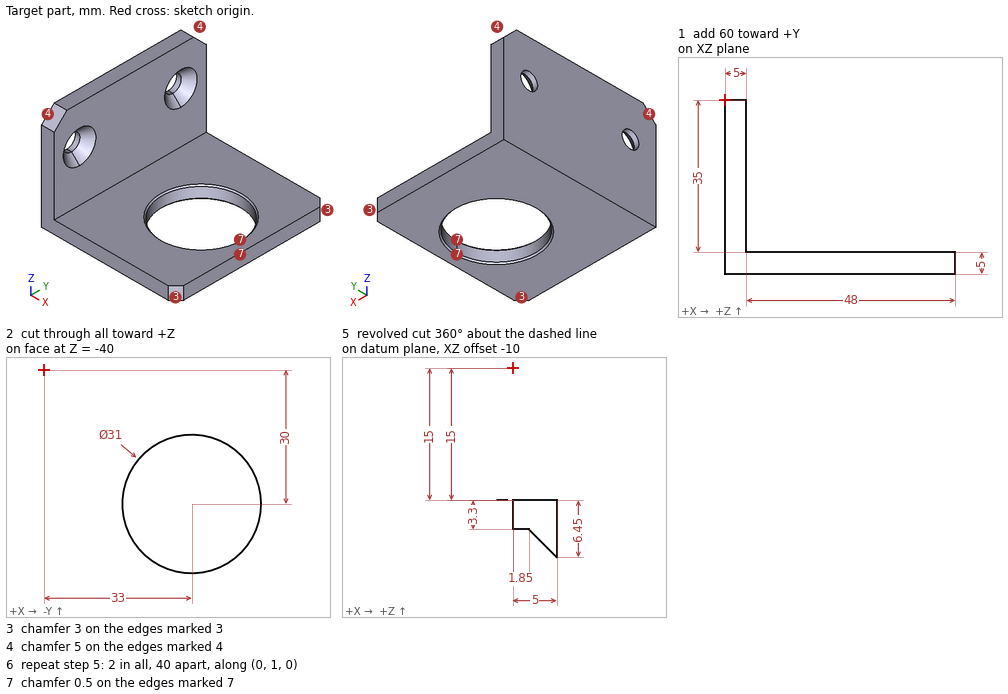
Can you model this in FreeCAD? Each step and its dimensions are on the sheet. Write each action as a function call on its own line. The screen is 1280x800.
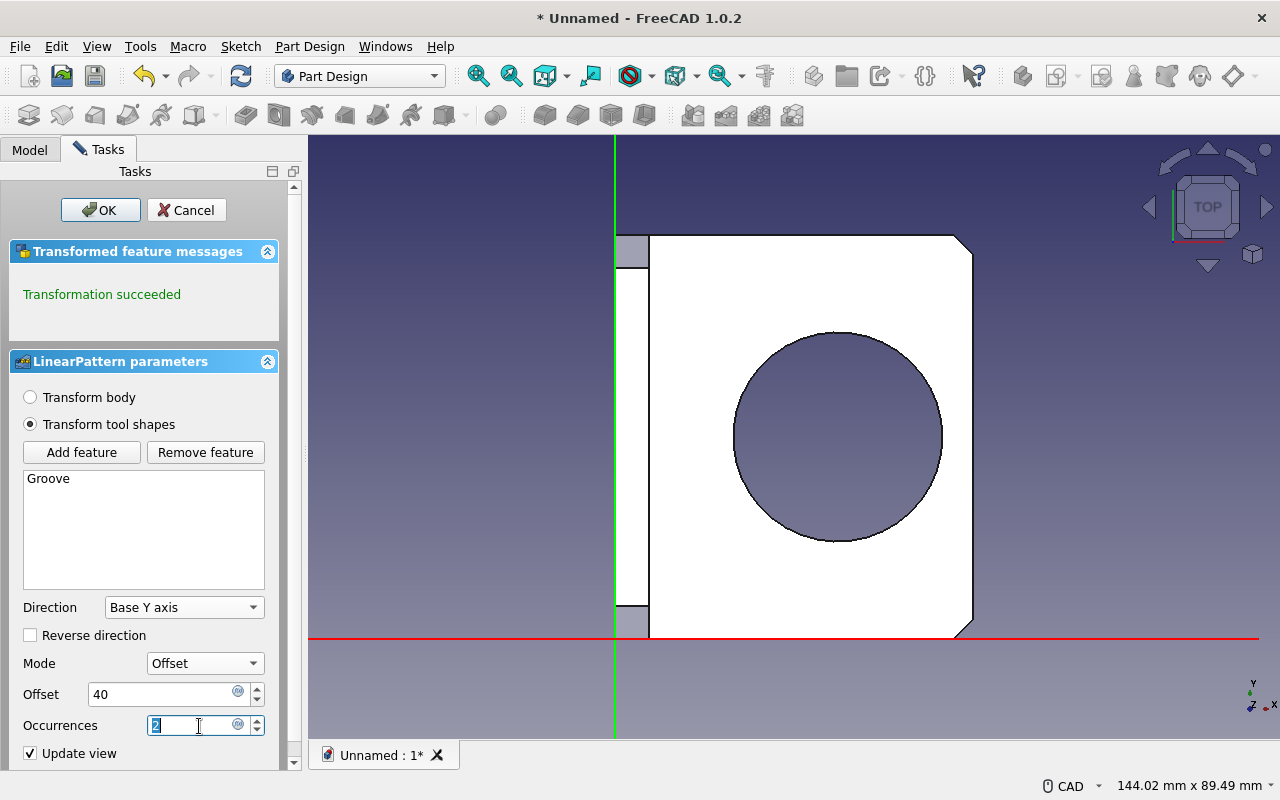
text(2)
key(Tab)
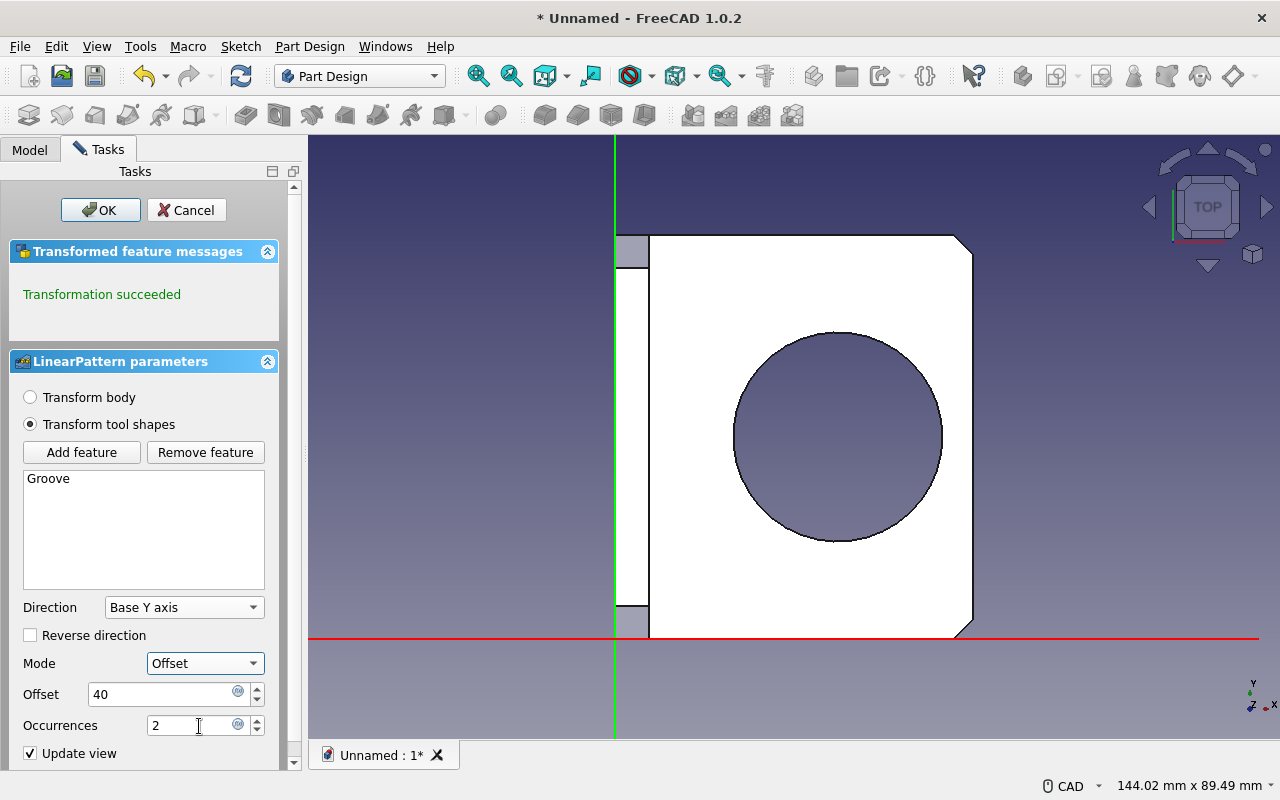
click(101, 210)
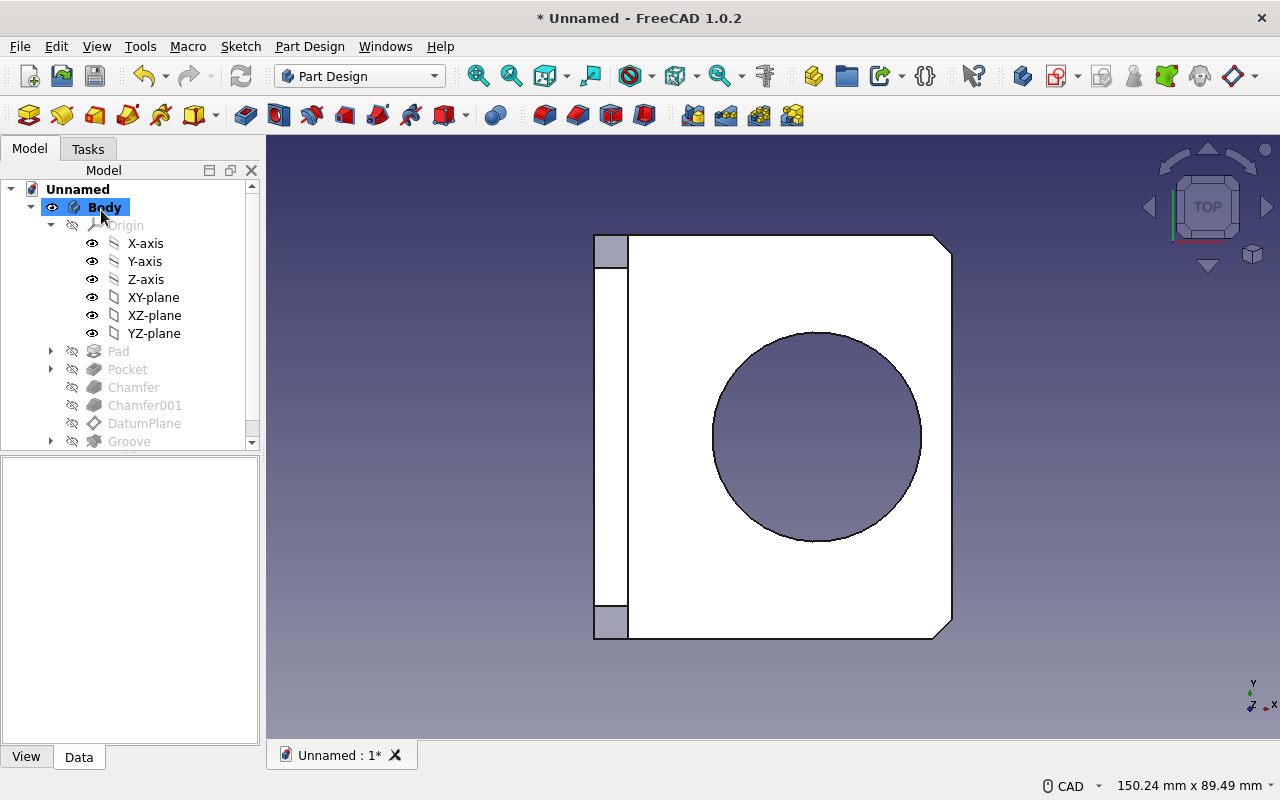
click(712, 436)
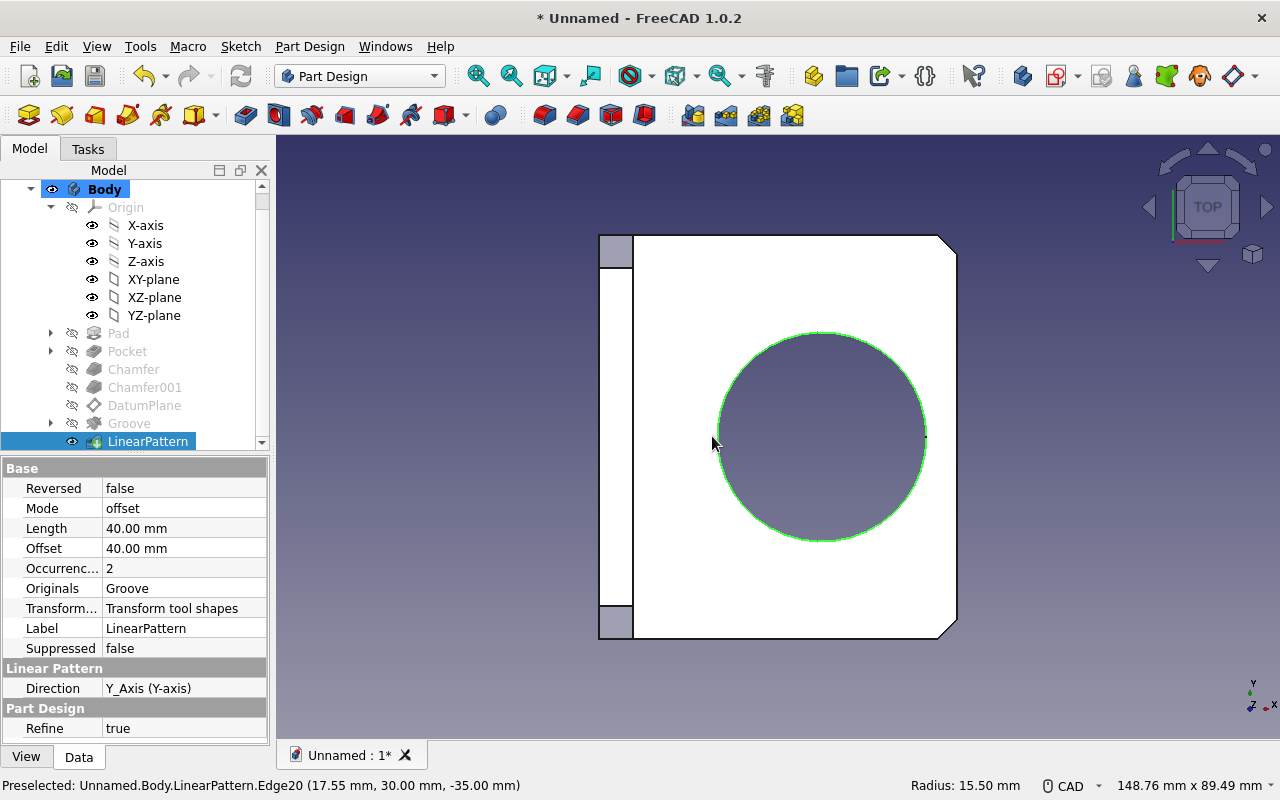
key(0)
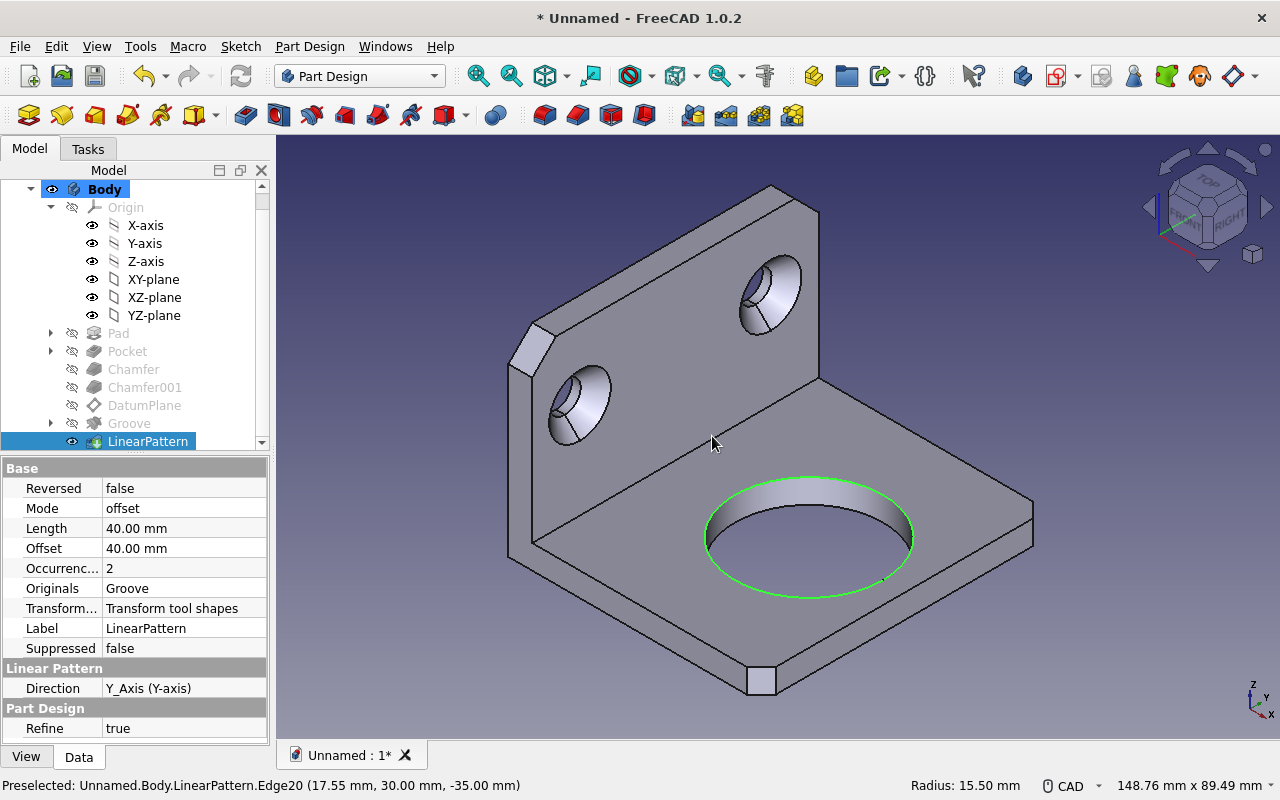
key(2)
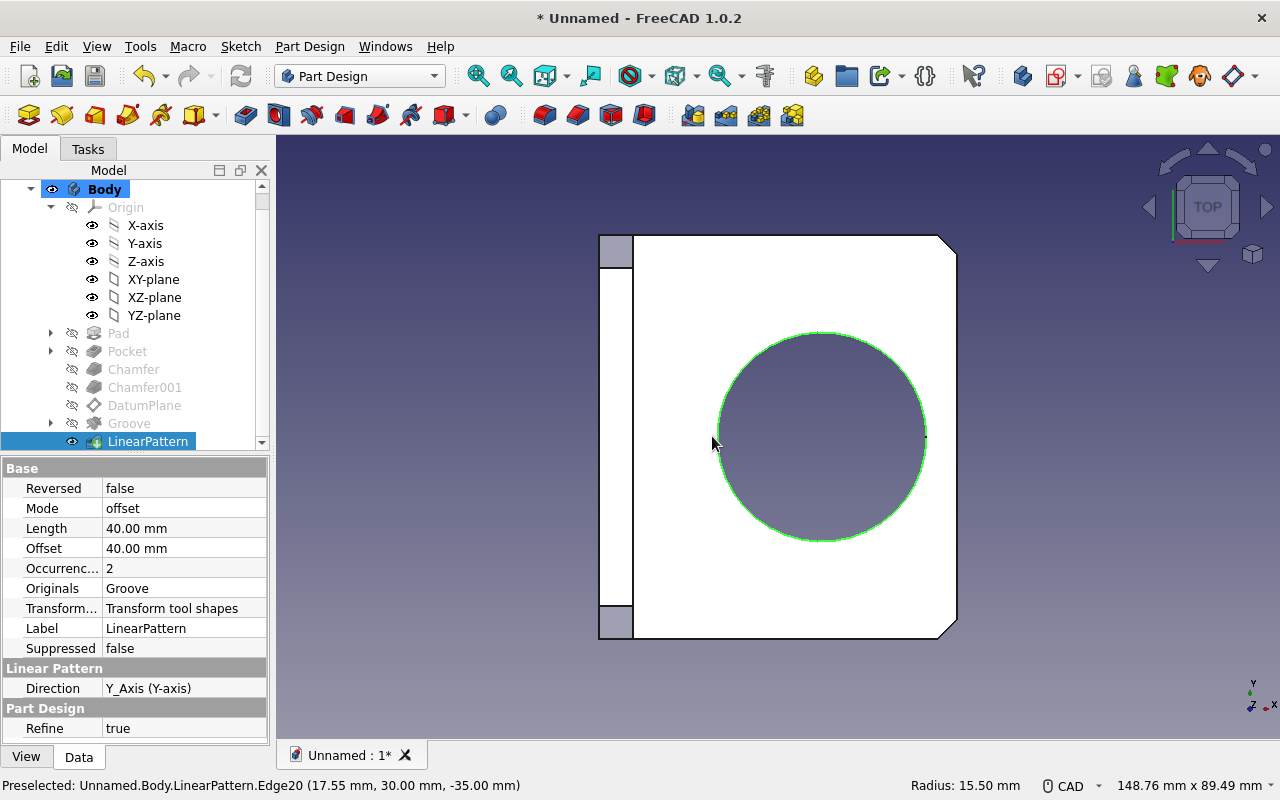
key(1)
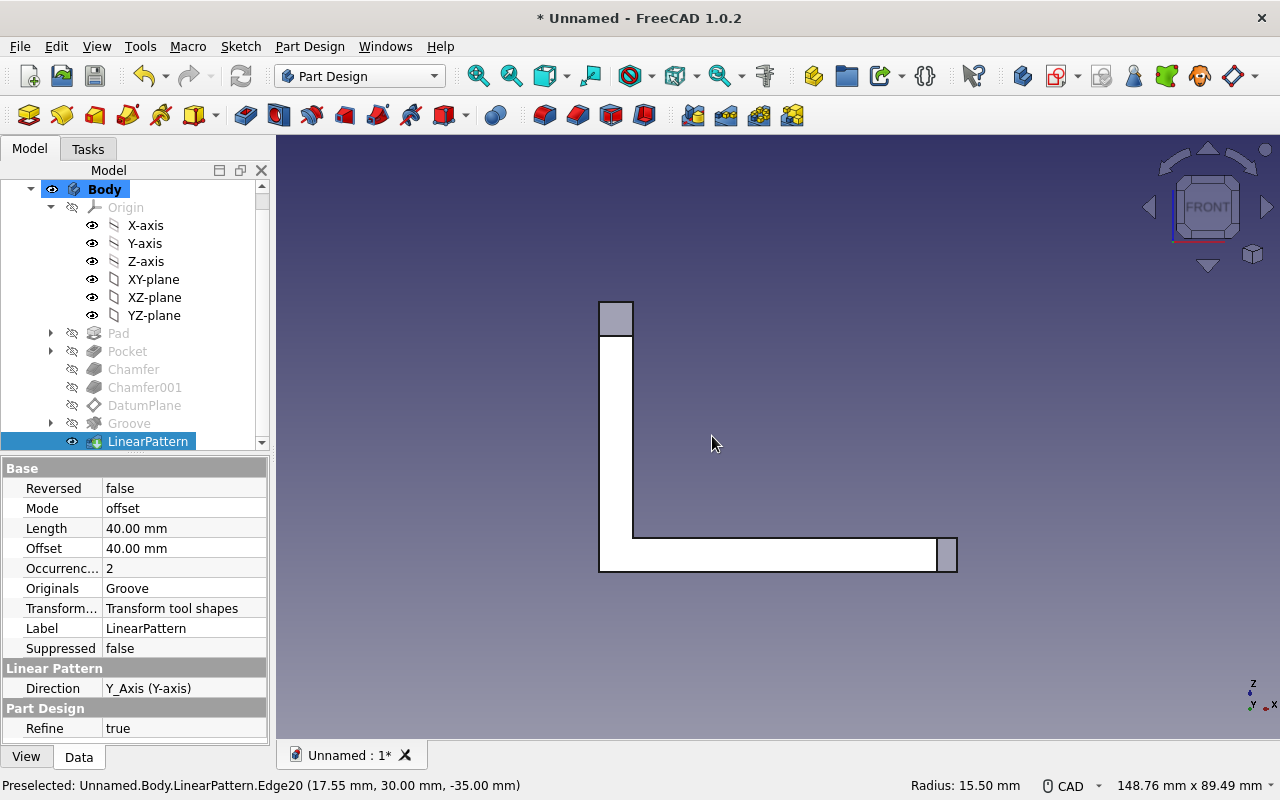
key(v)
key(f)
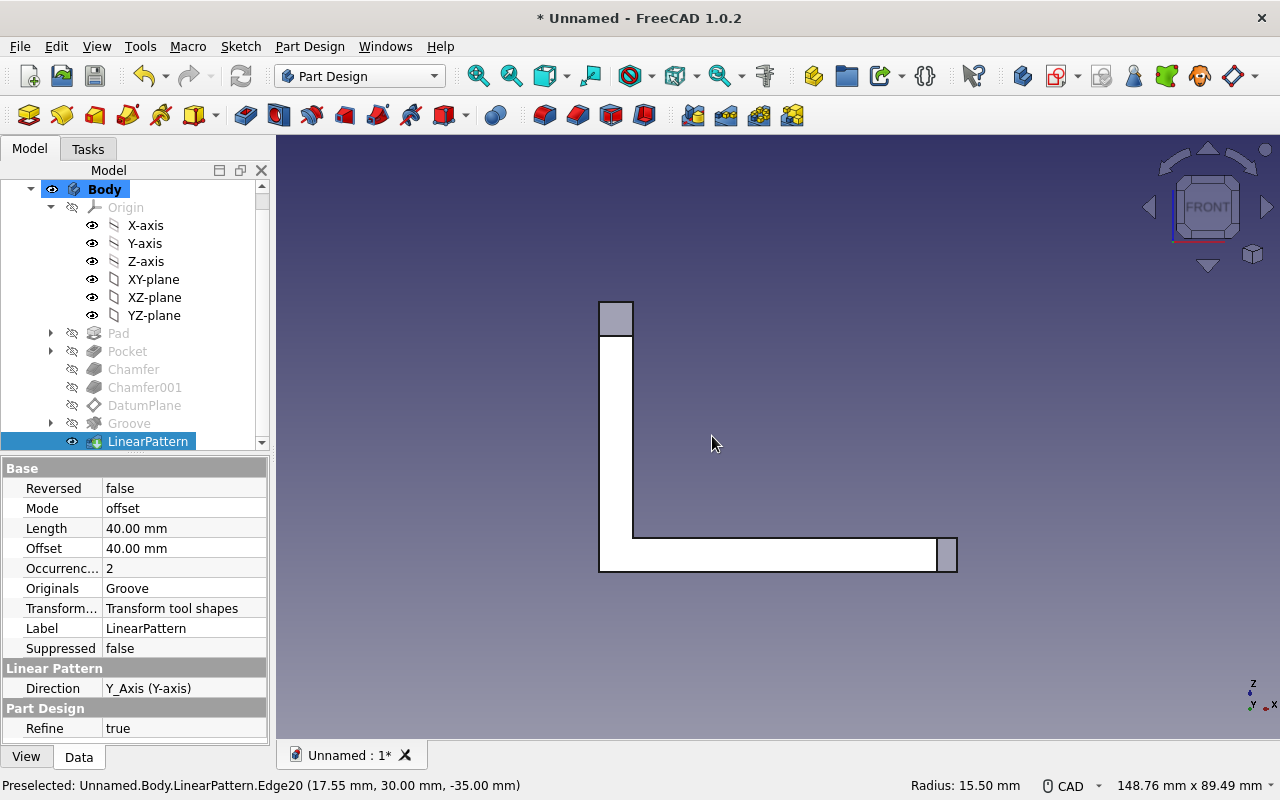
key(3)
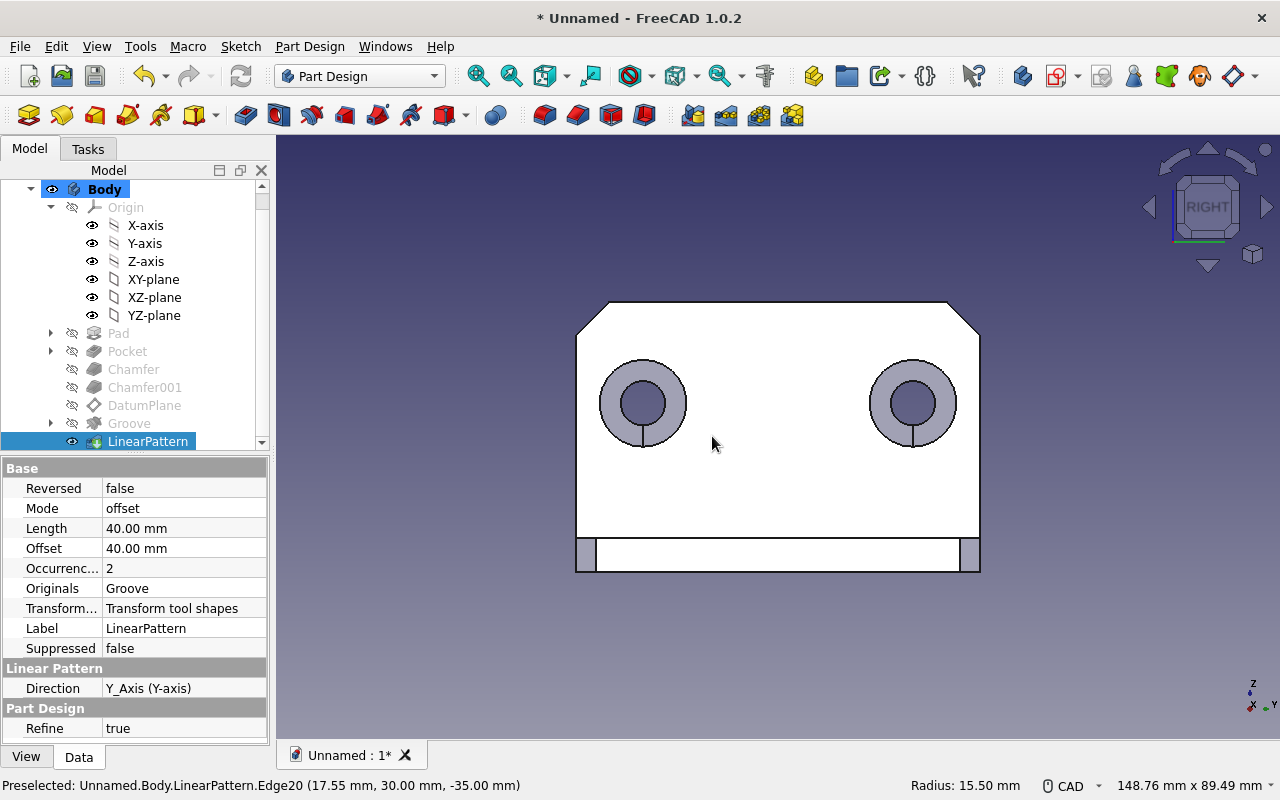
key(v)
key(f)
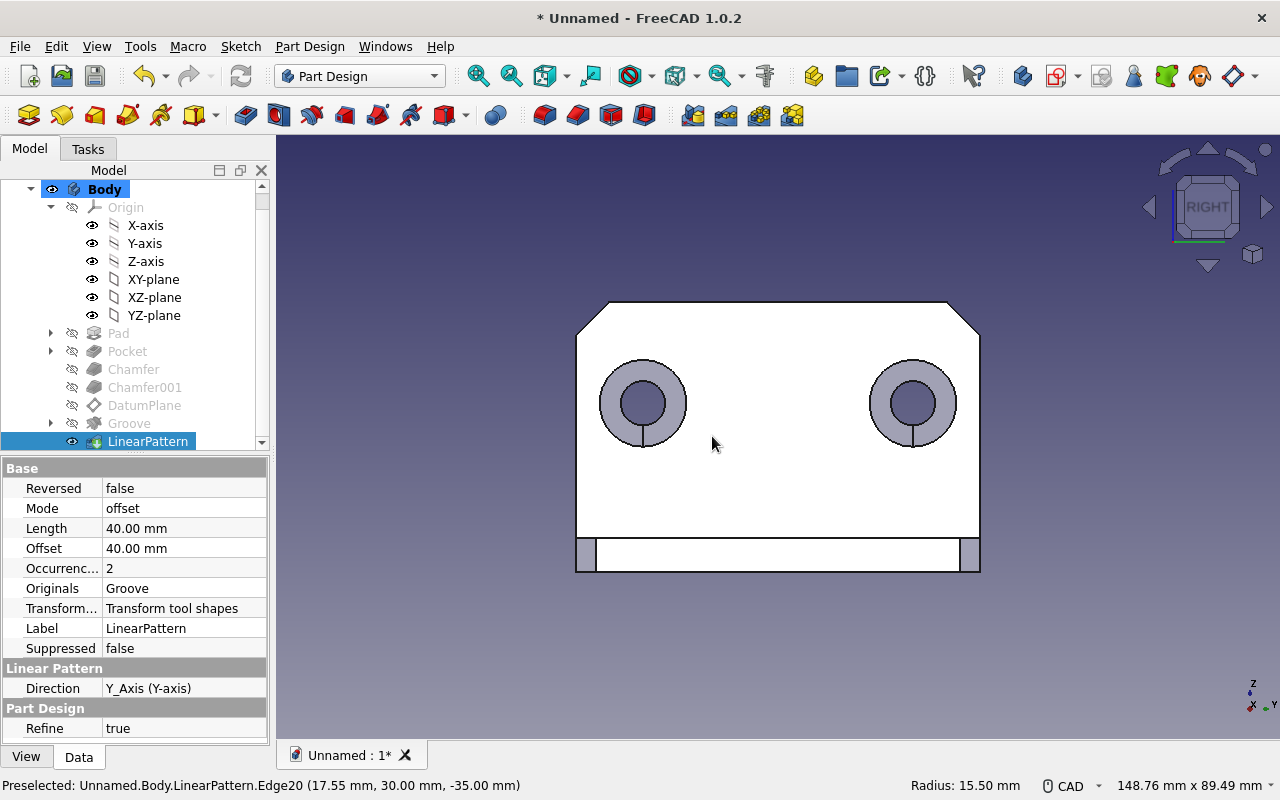
key(5)